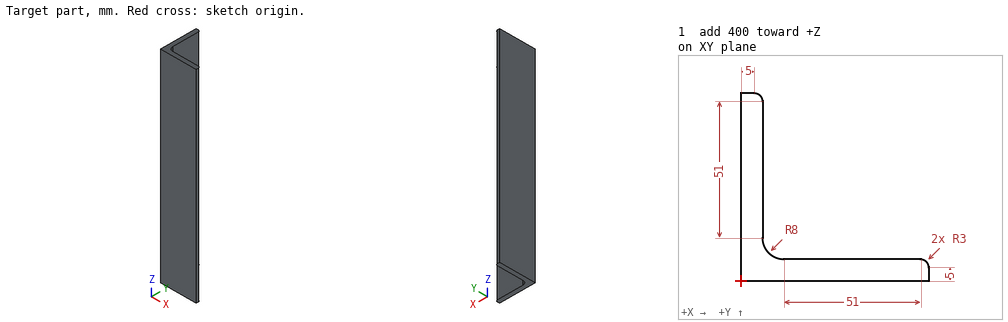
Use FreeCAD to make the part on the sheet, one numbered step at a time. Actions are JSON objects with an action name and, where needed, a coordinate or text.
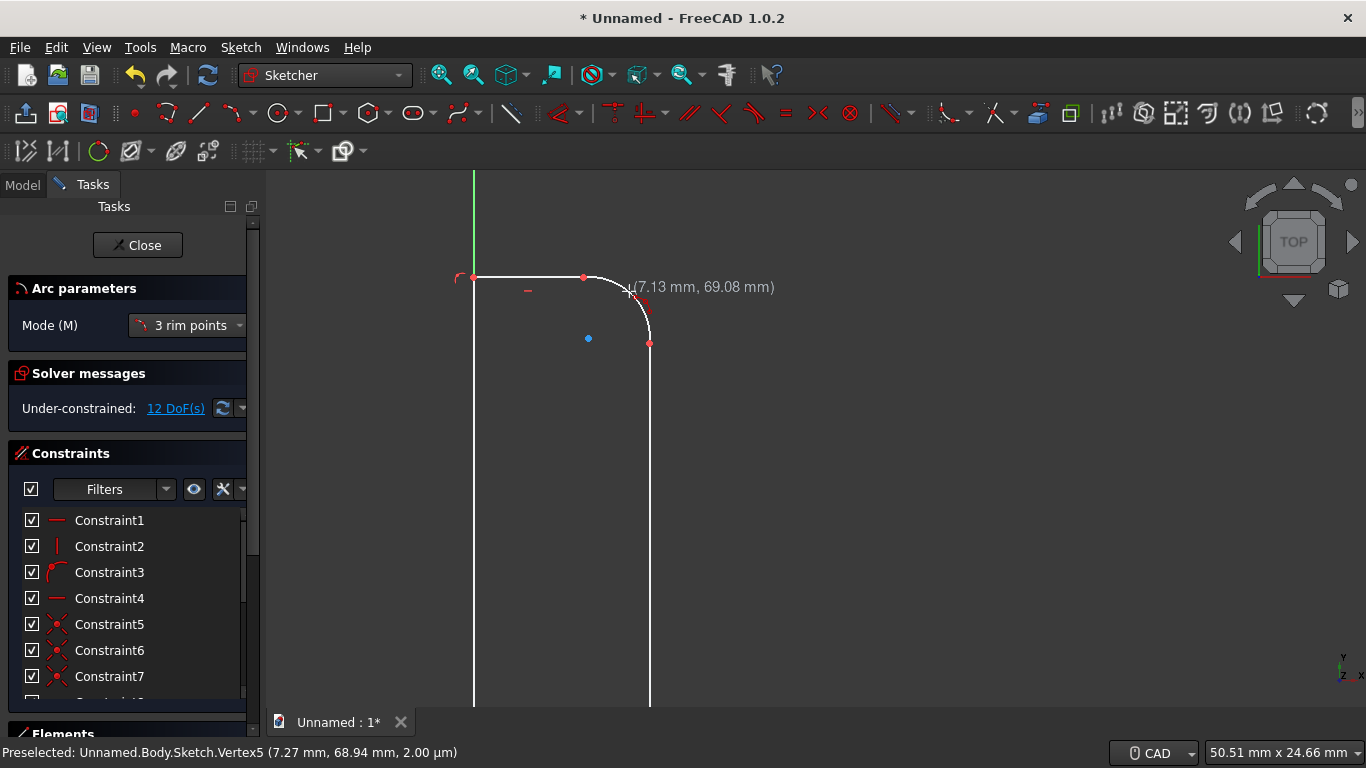
{"action": "scroll", "coordinate": [624, 288], "scroll_direction": "down", "scroll_amount": 8}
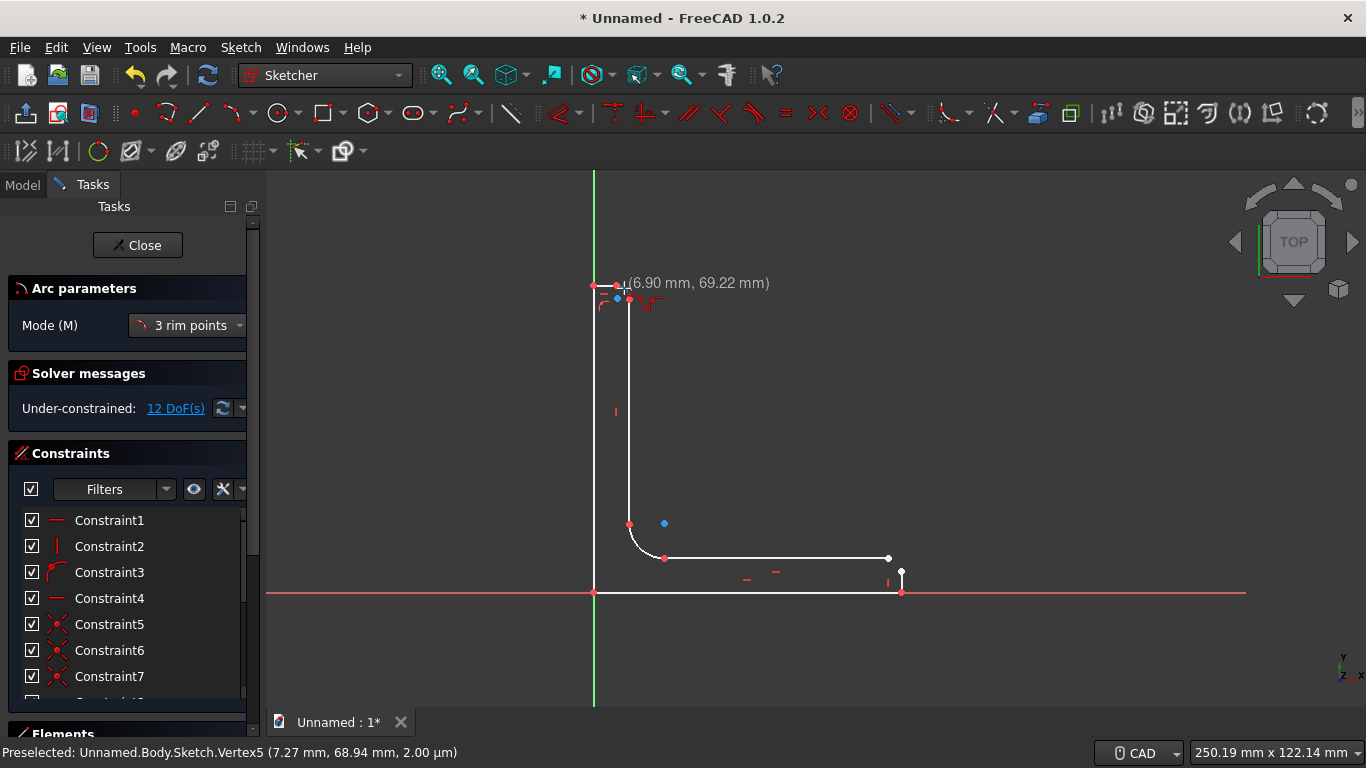
{"action": "scroll", "coordinate": [902, 571], "scroll_direction": "up", "scroll_amount": 2}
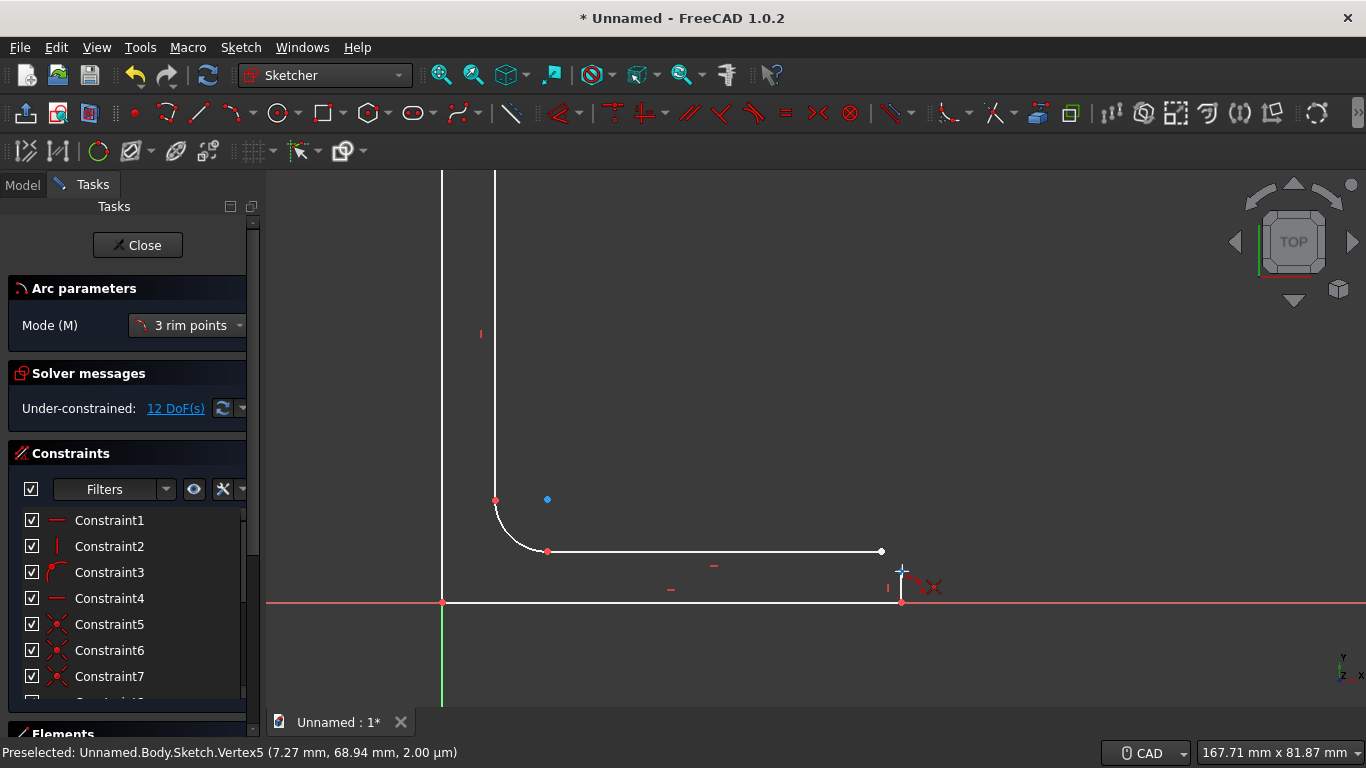
{"action": "left_click", "coordinate": [901, 572]}
{"action": "left_click", "coordinate": [881, 552]}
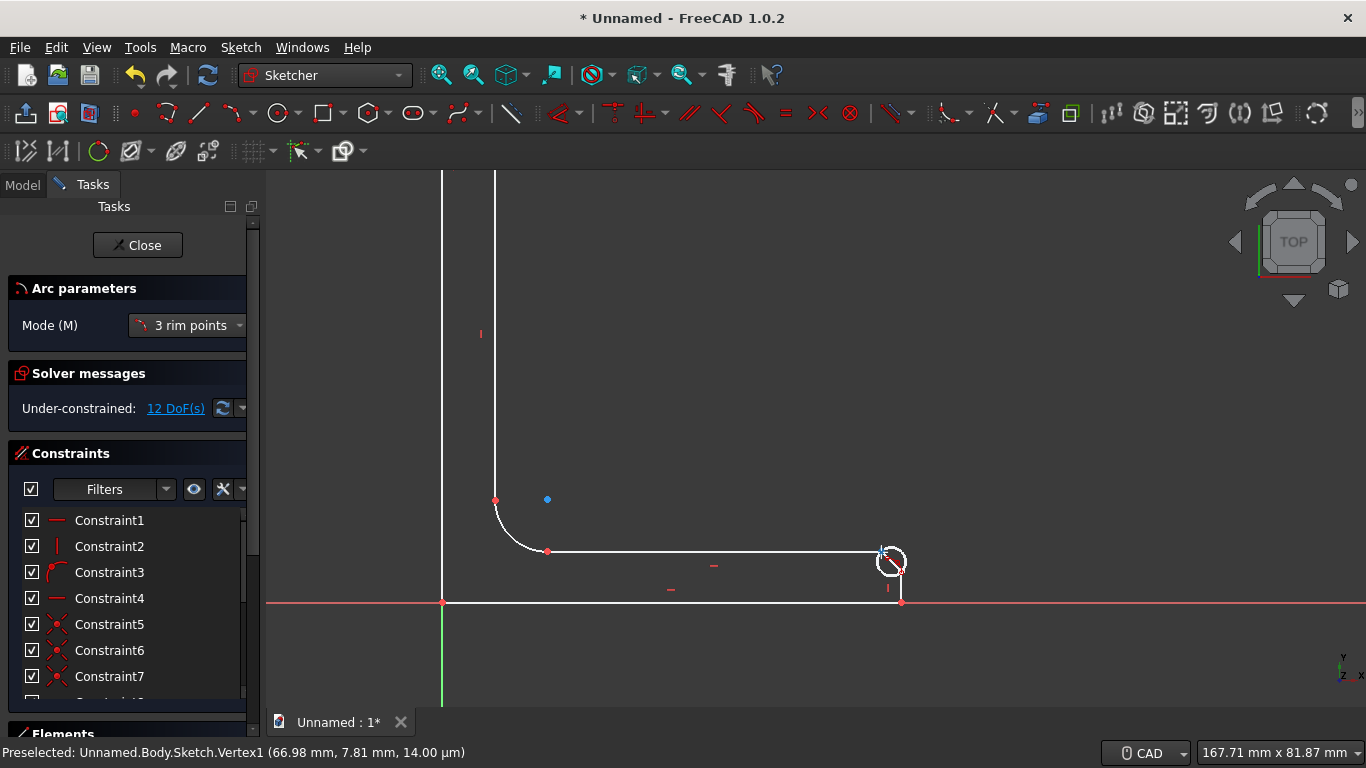
{"action": "scroll", "coordinate": [895, 556], "scroll_direction": "up", "scroll_amount": 6}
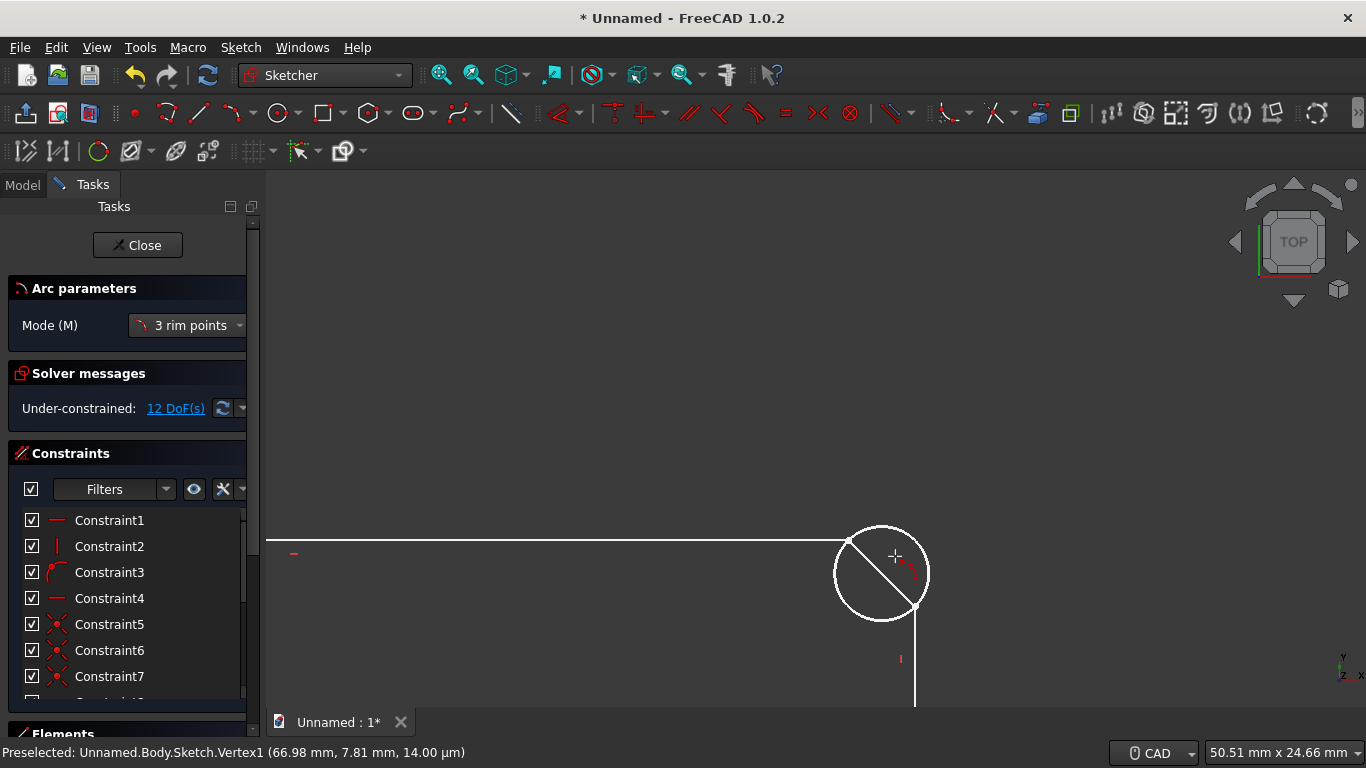
{"action": "left_click", "coordinate": [895, 555]}
{"action": "key", "text": "Escape"}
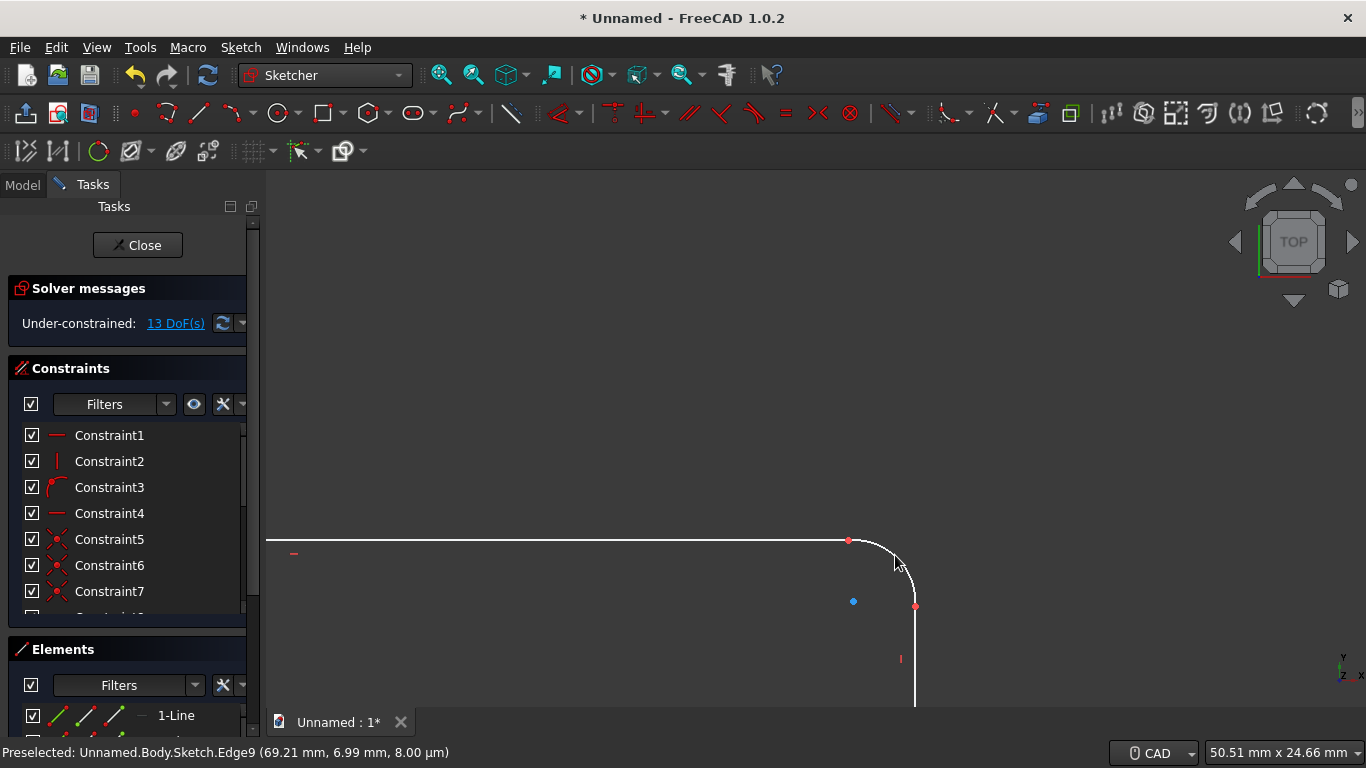
{"action": "scroll", "coordinate": [898, 563], "scroll_direction": "down", "scroll_amount": 8}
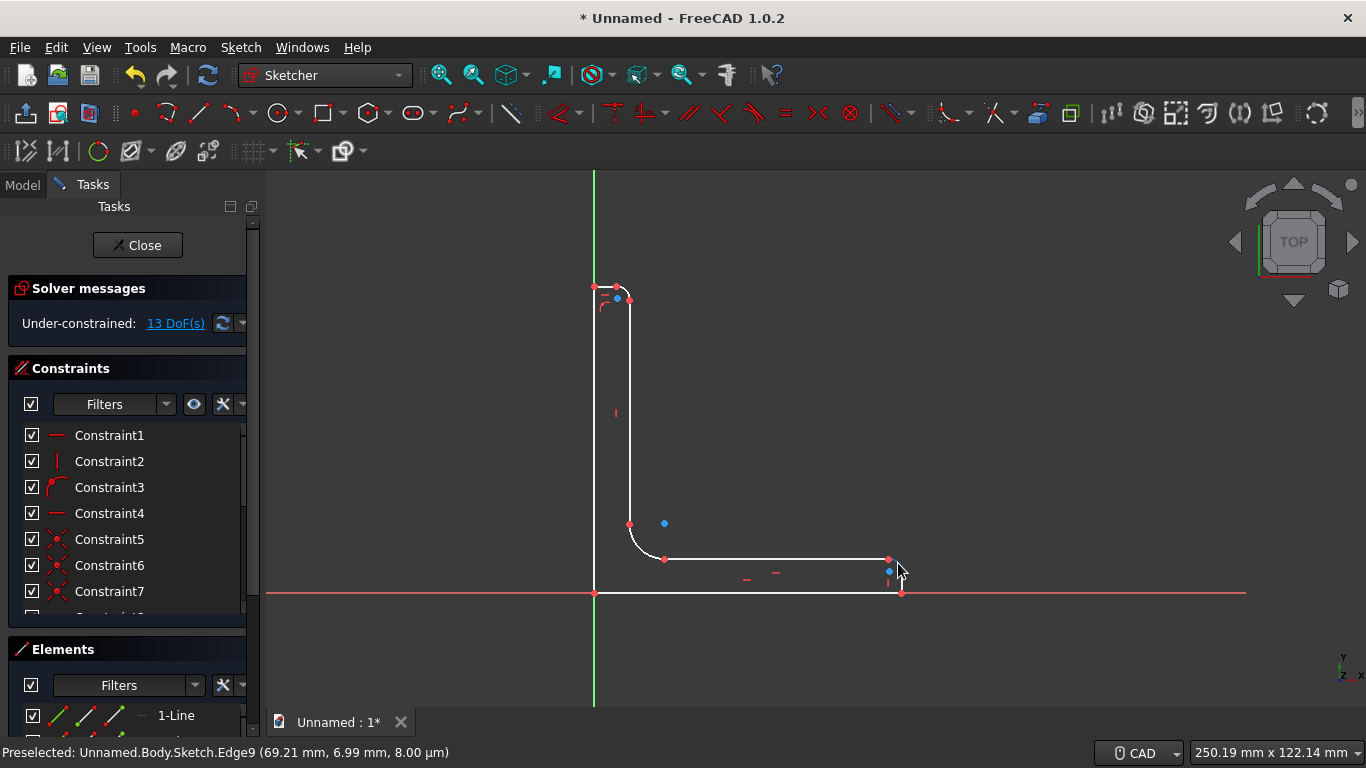
{"action": "left_click", "coordinate": [821, 559]}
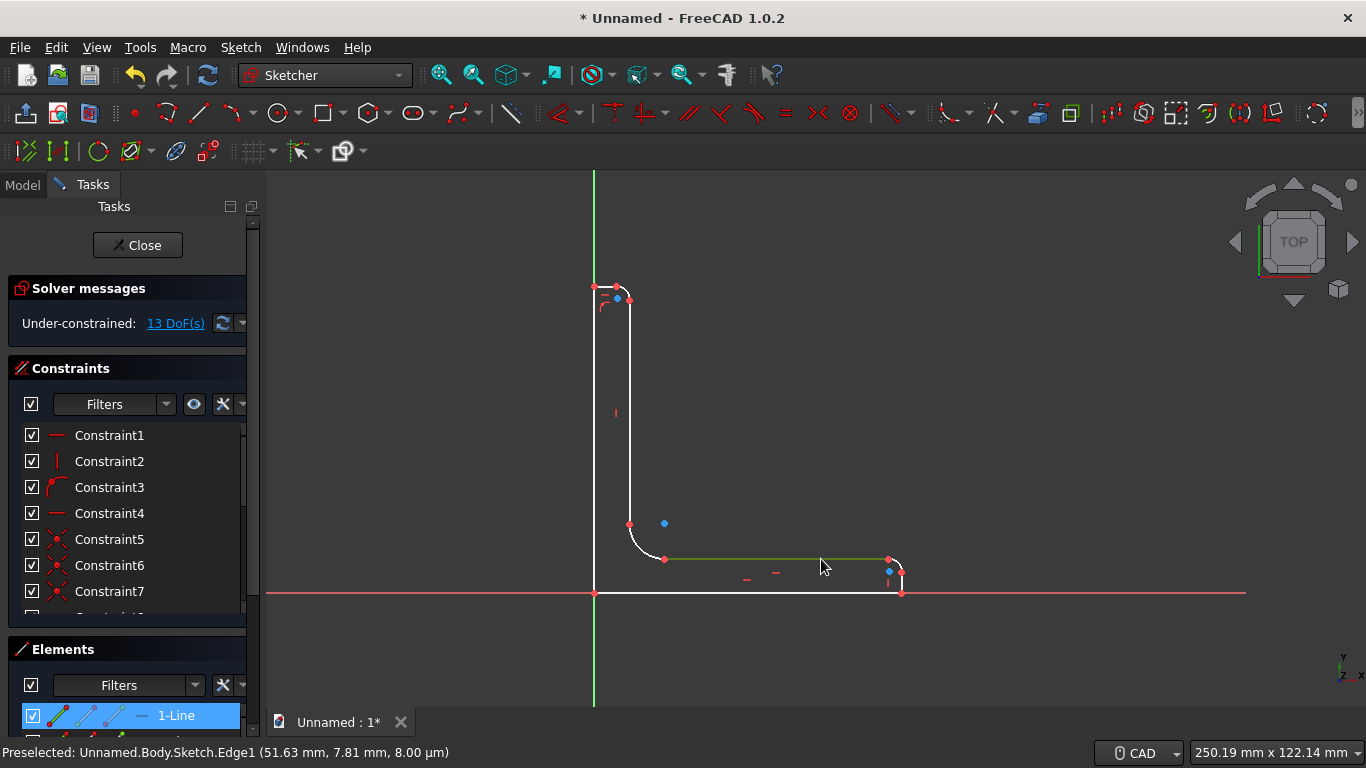
{"action": "left_click", "coordinate": [634, 540]}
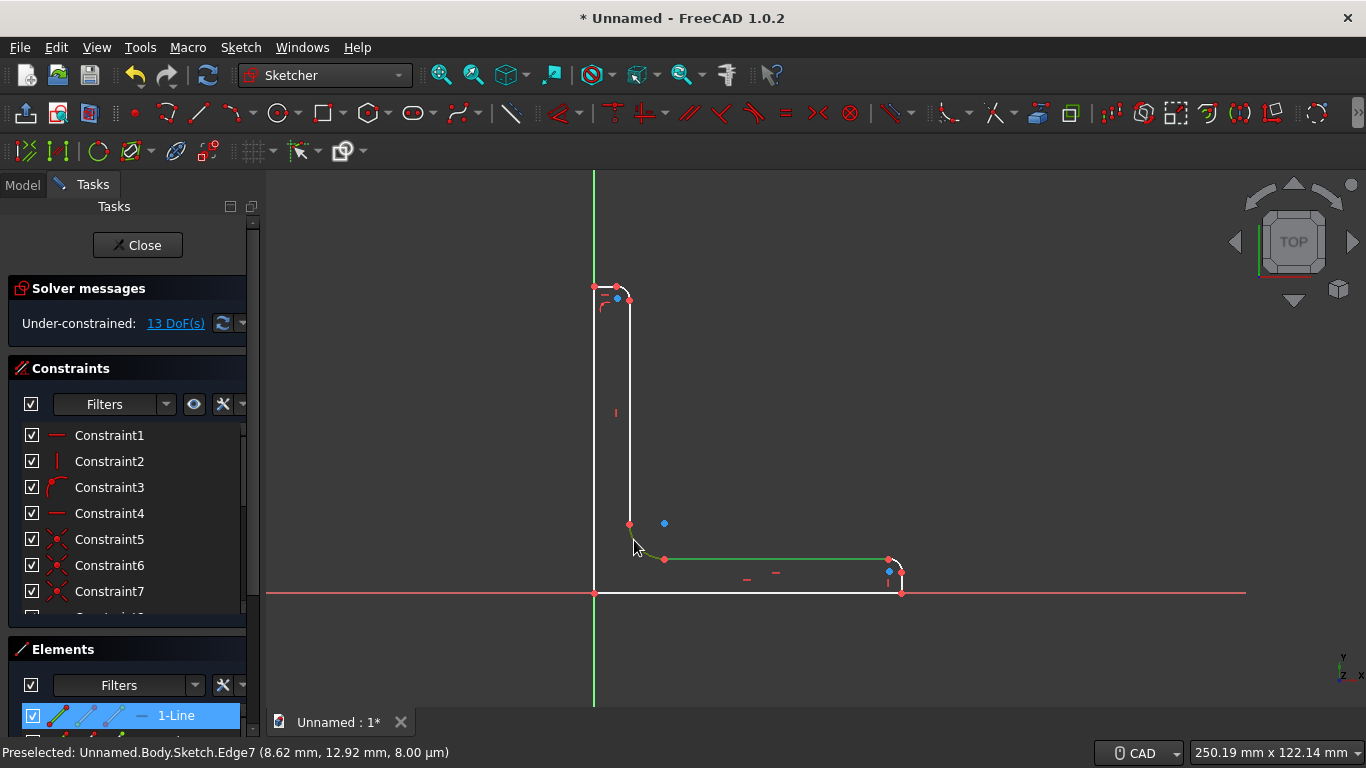
{"action": "left_click", "coordinate": [754, 114]}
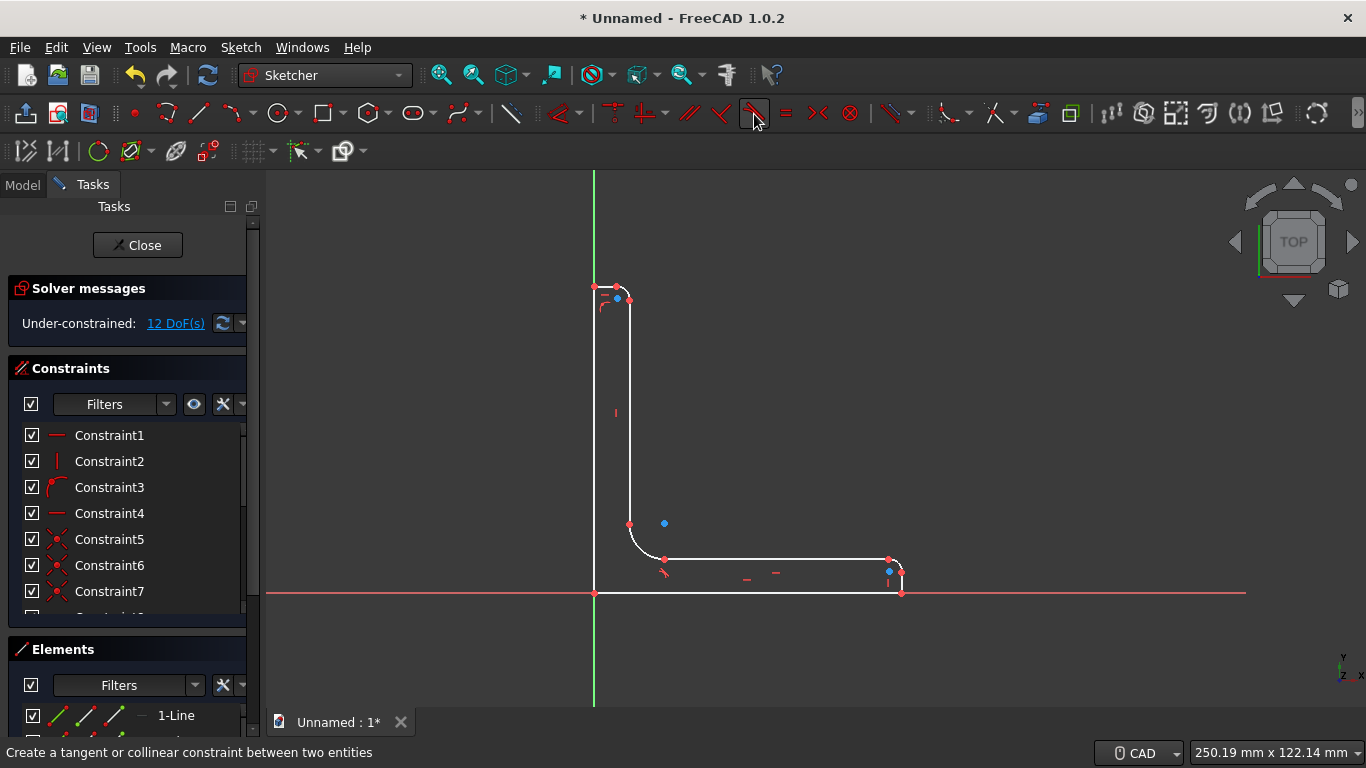
{"action": "left_click", "coordinate": [821, 559]}